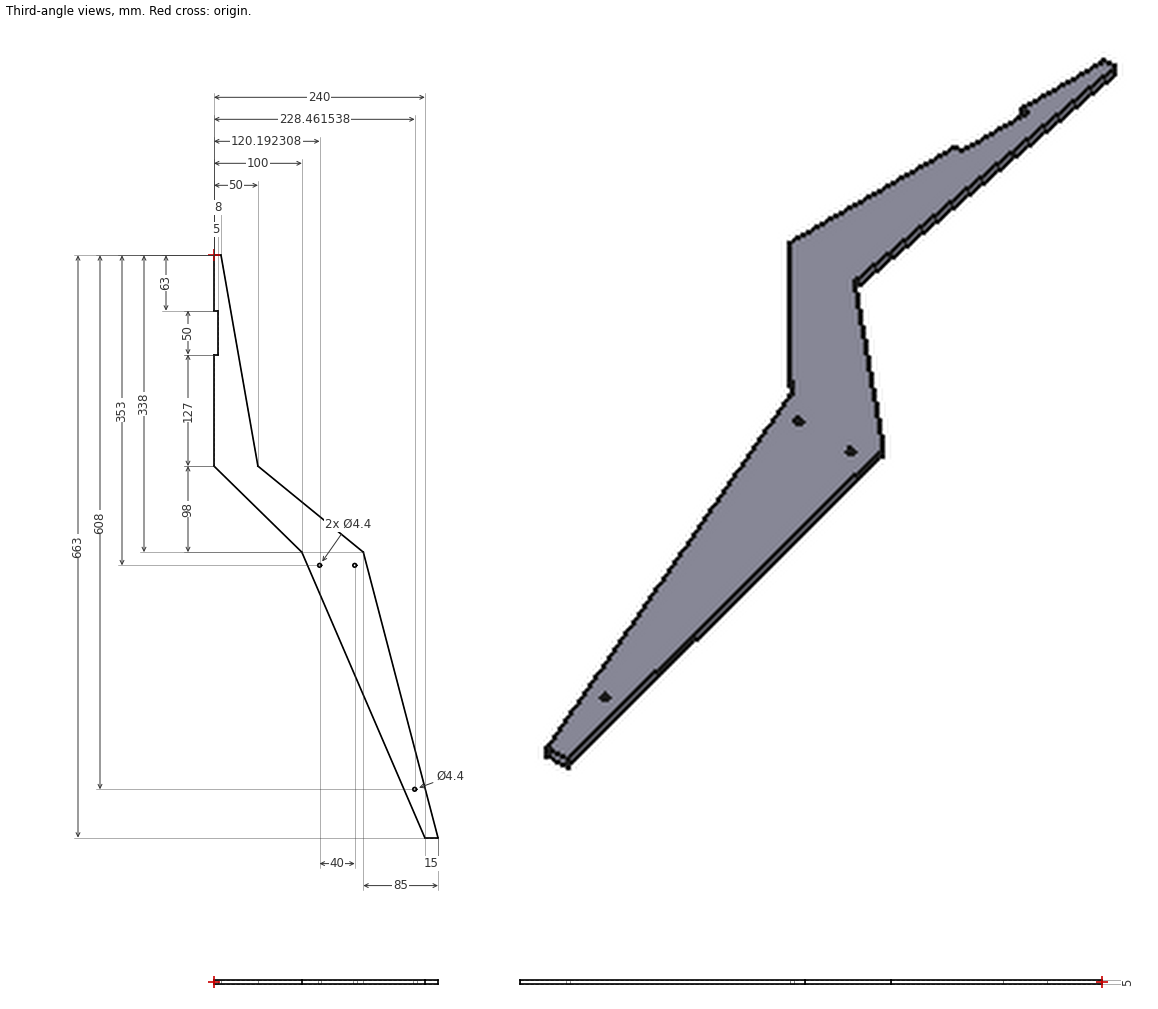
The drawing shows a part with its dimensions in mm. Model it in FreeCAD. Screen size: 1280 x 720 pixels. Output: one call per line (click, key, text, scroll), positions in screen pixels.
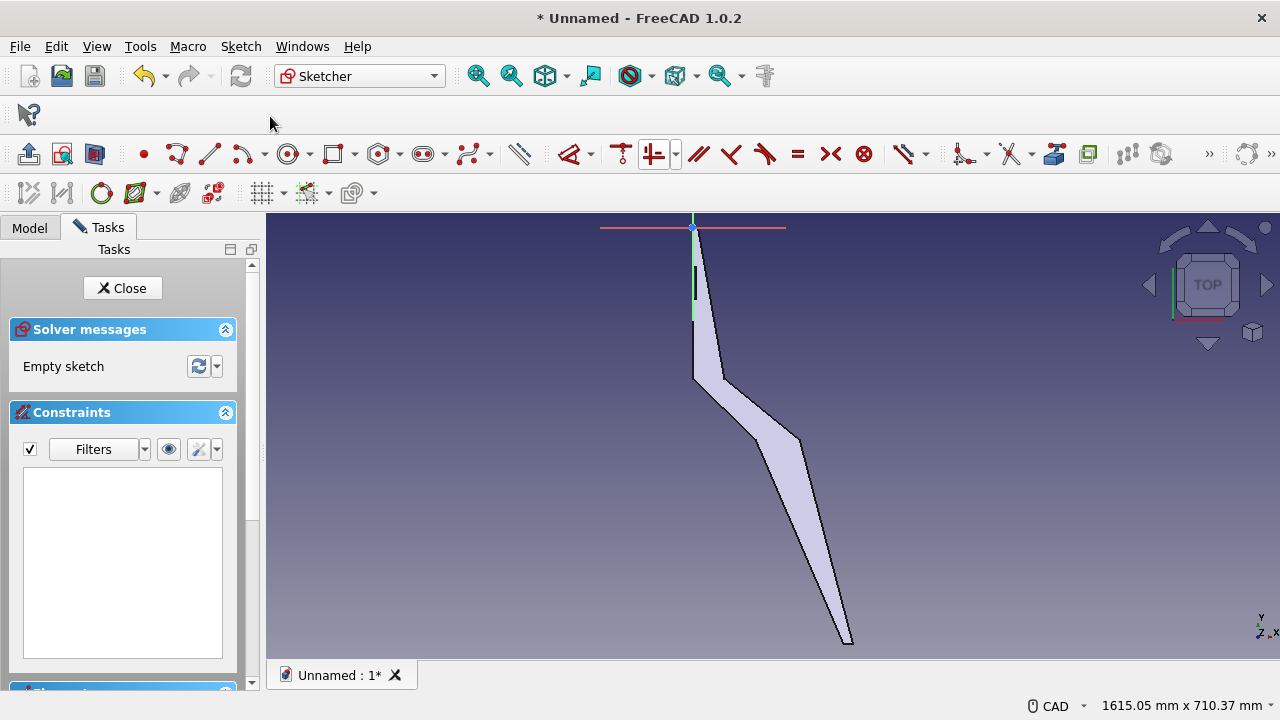
scroll(785, 450, up, 15)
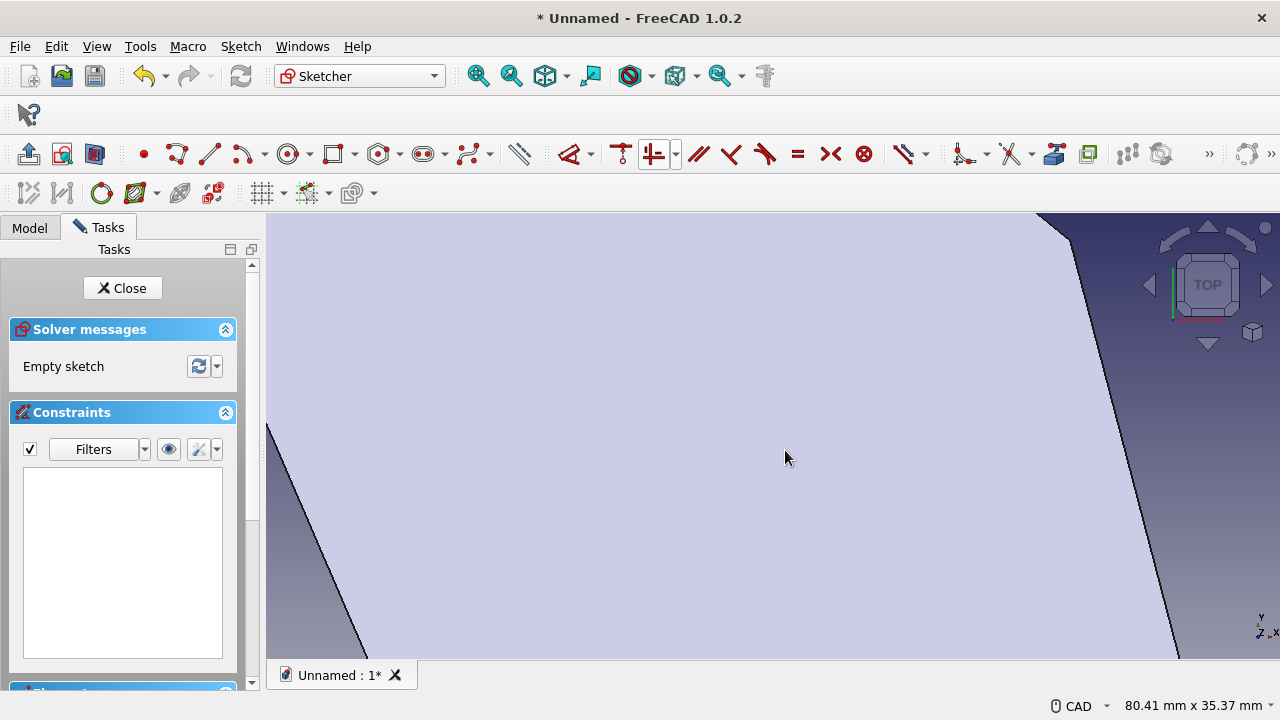
click(288, 154)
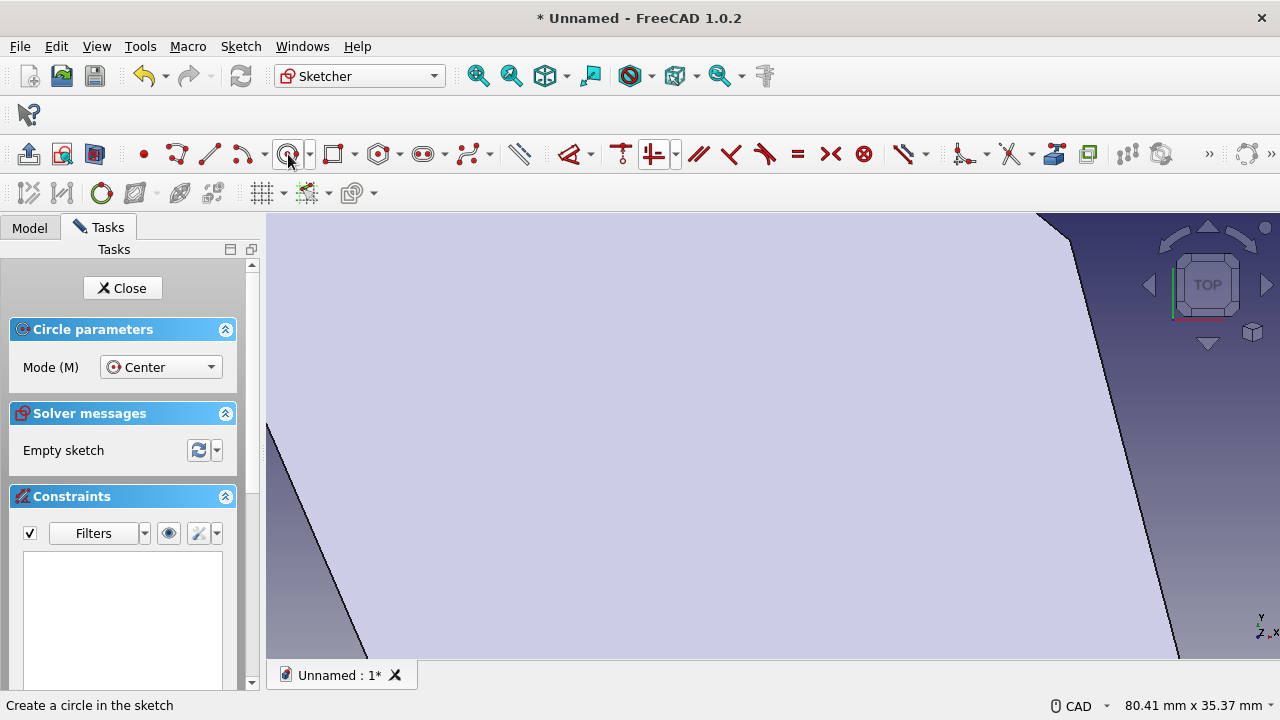
click(442, 430)
click(462, 410)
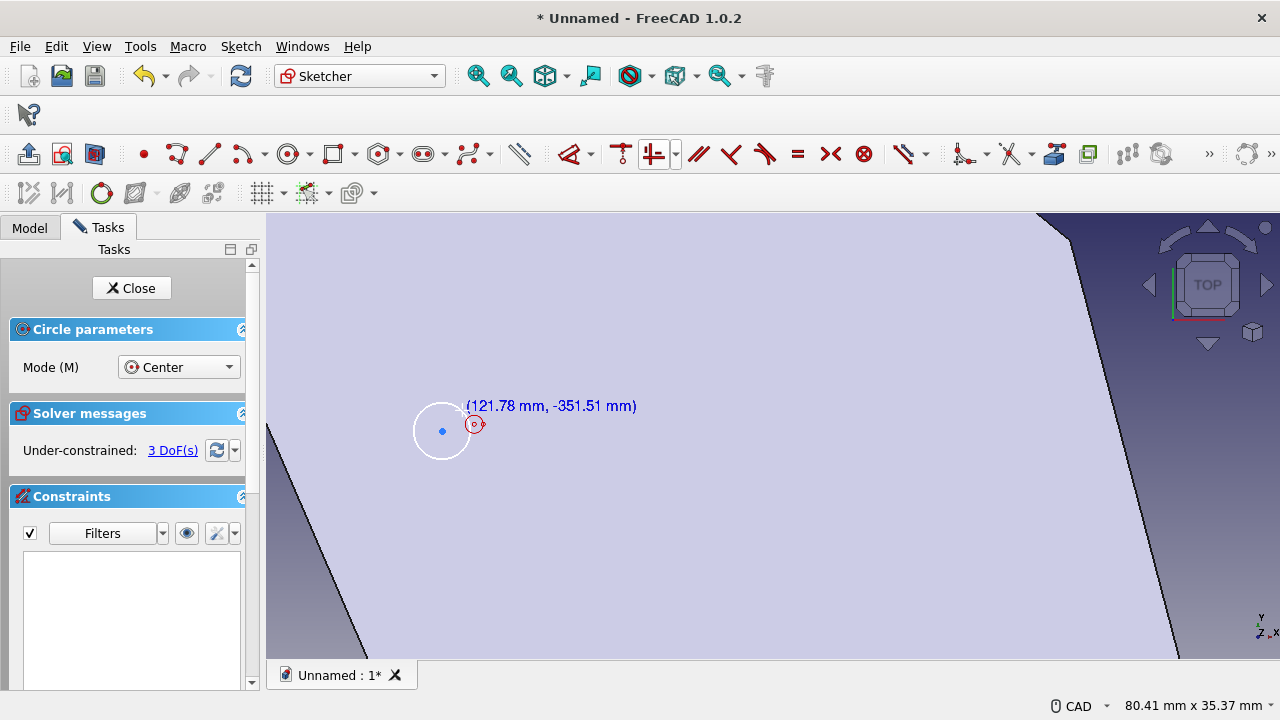
click(946, 430)
click(966, 410)
key(Escape)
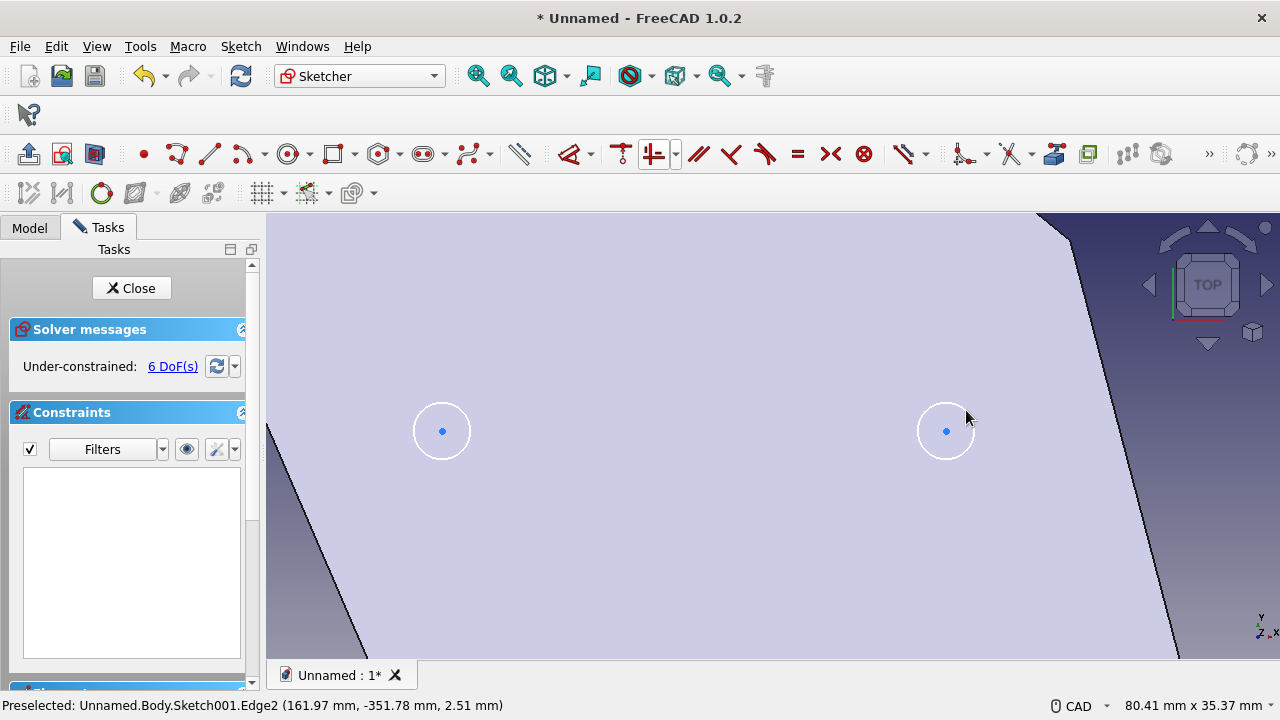
click(462, 411)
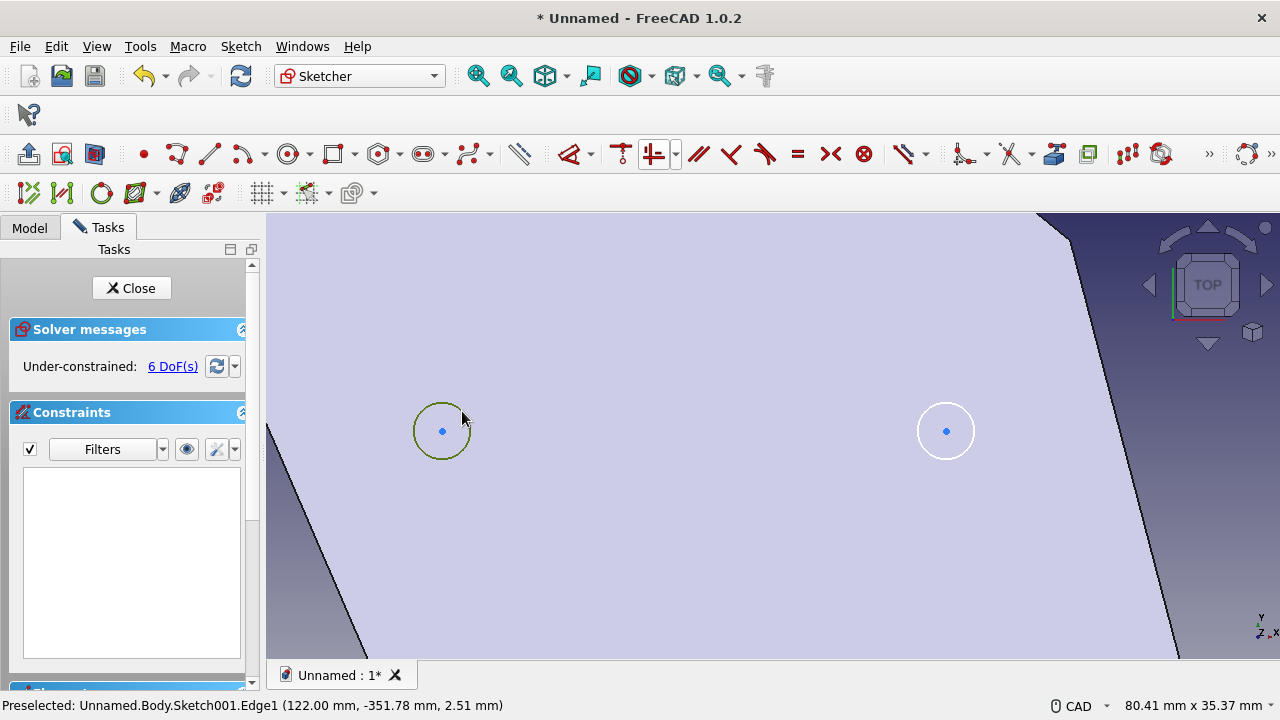
click(966, 411)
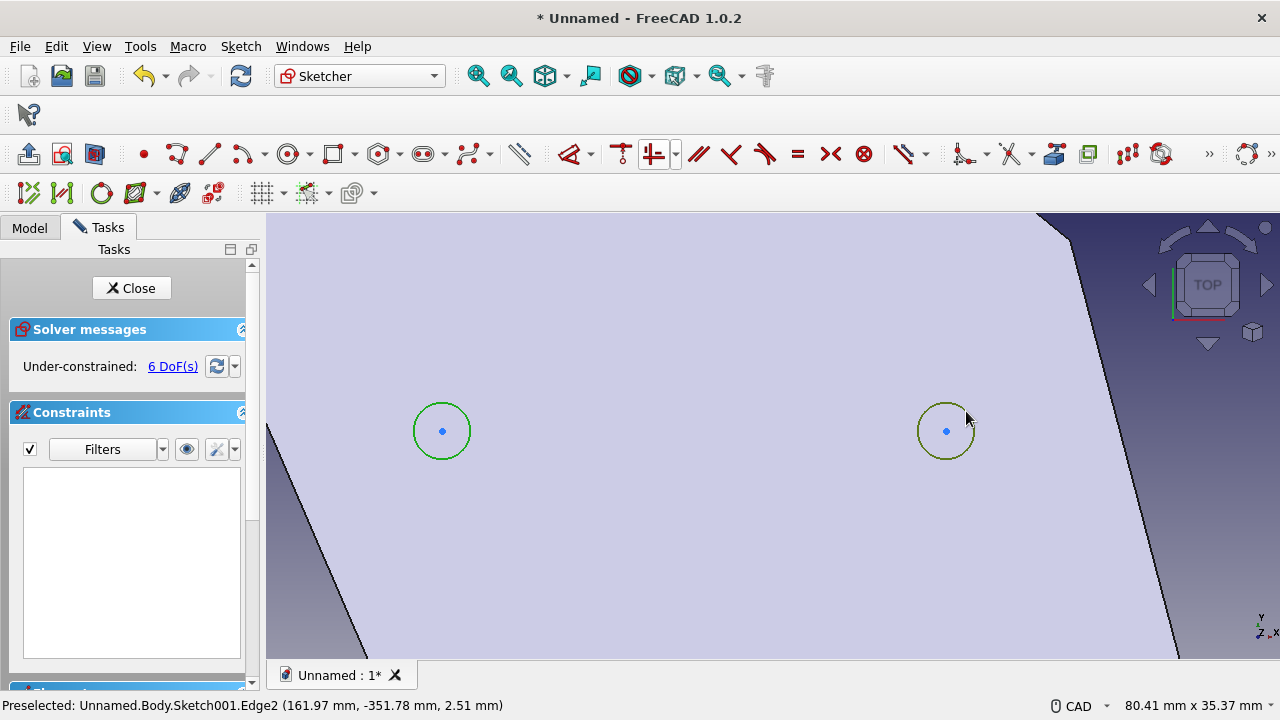
click(798, 154)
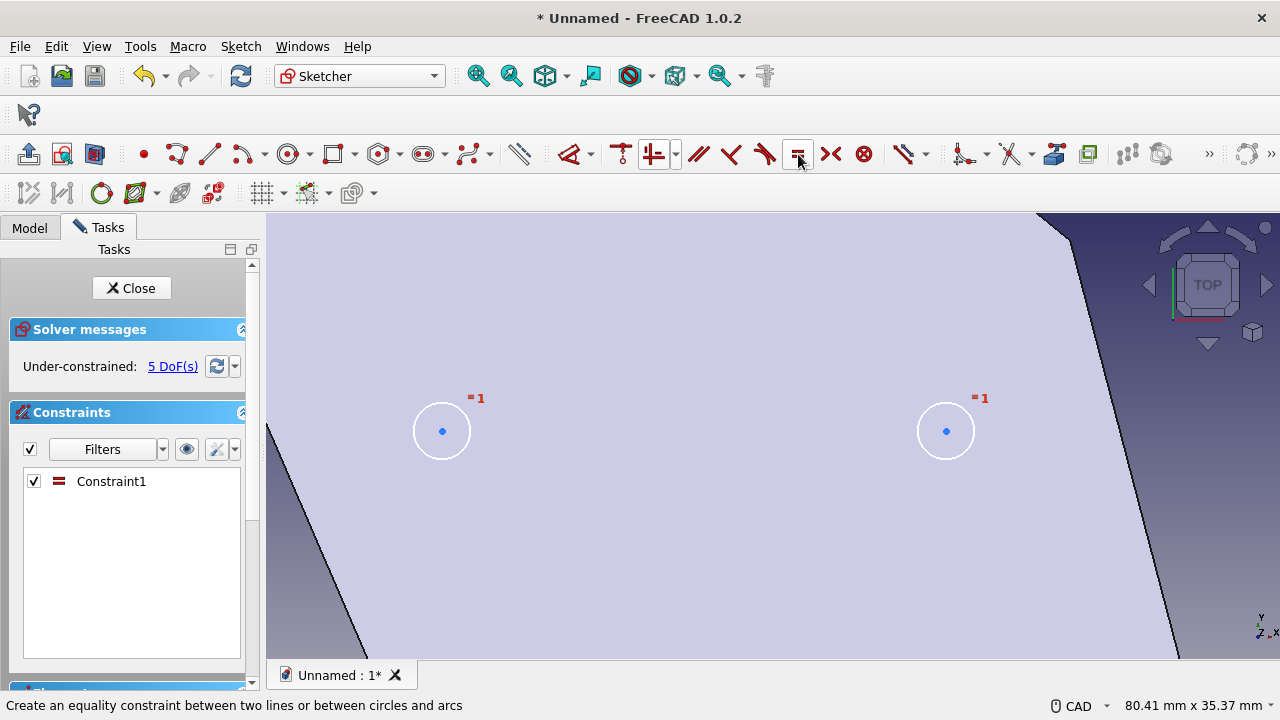
click(442, 431)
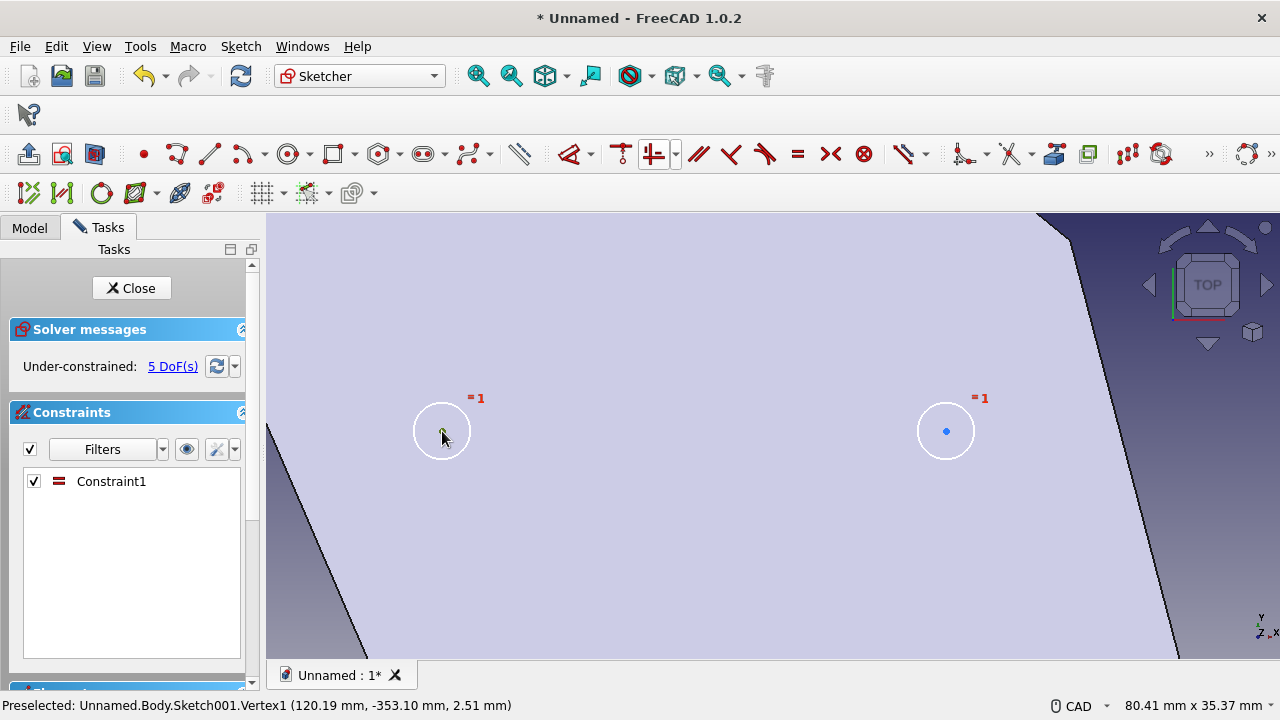
click(946, 431)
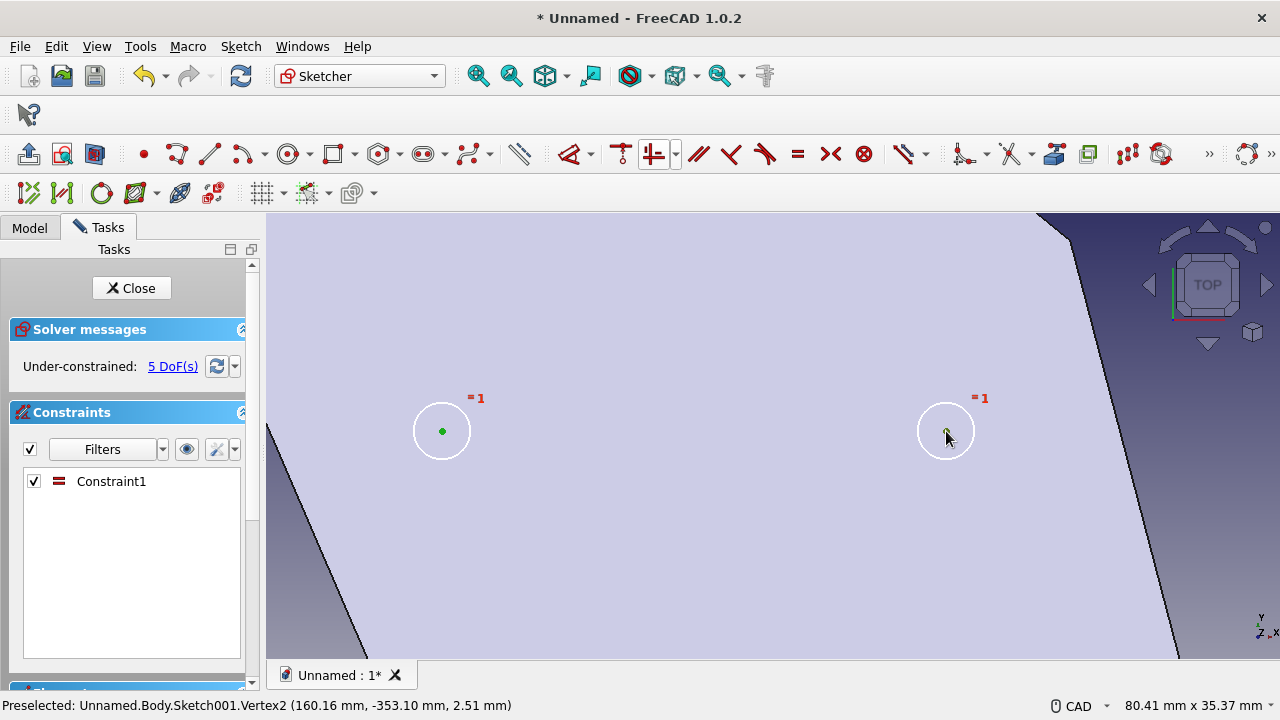
key(h)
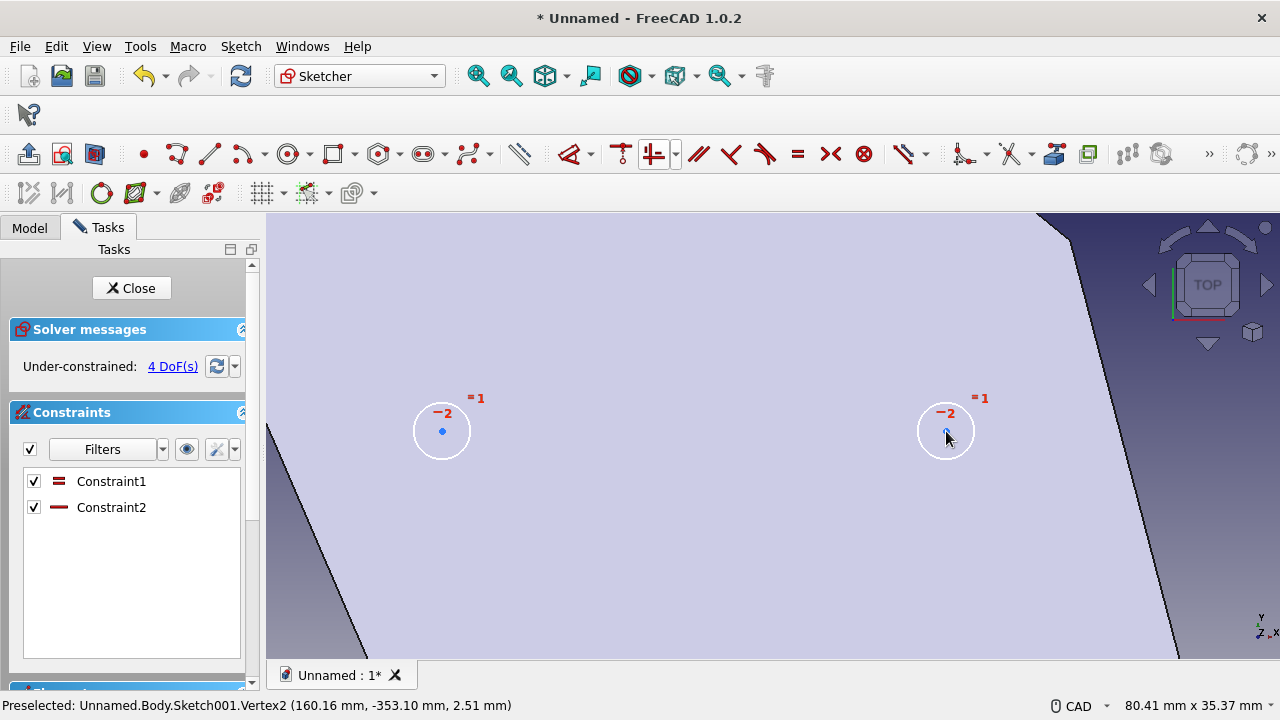
click(568, 154)